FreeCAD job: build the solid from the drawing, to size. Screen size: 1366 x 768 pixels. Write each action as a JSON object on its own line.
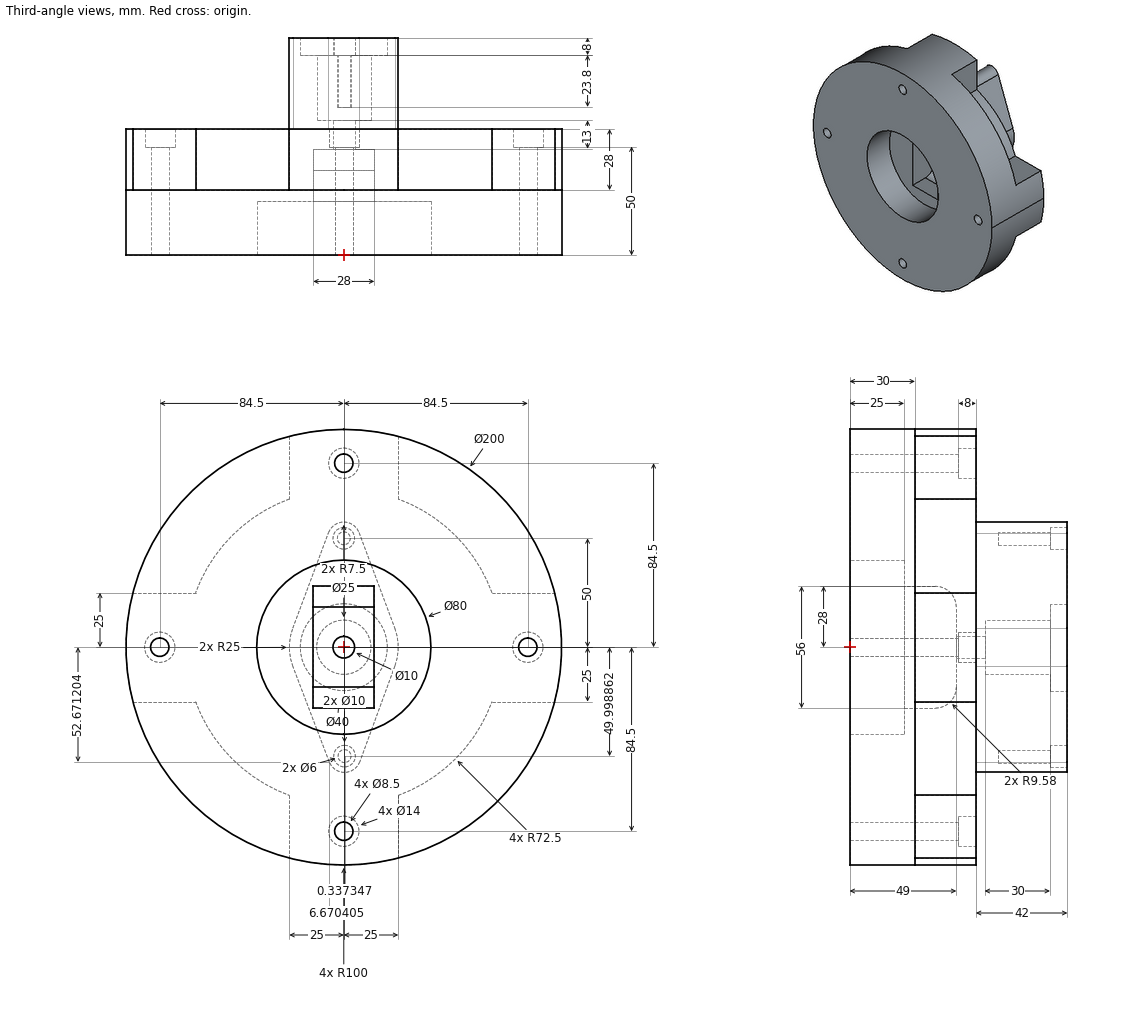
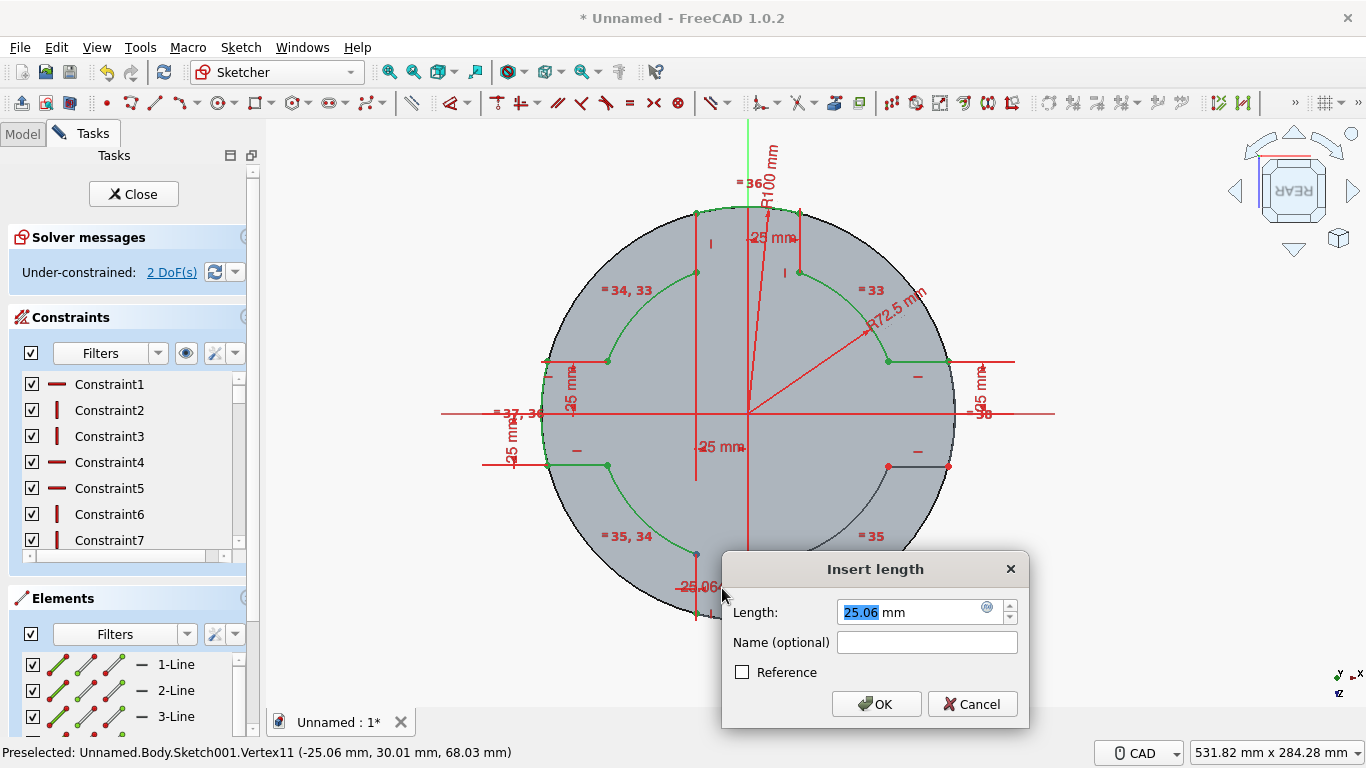
{"action": "type", "text": "25"}
{"action": "key", "text": "Return"}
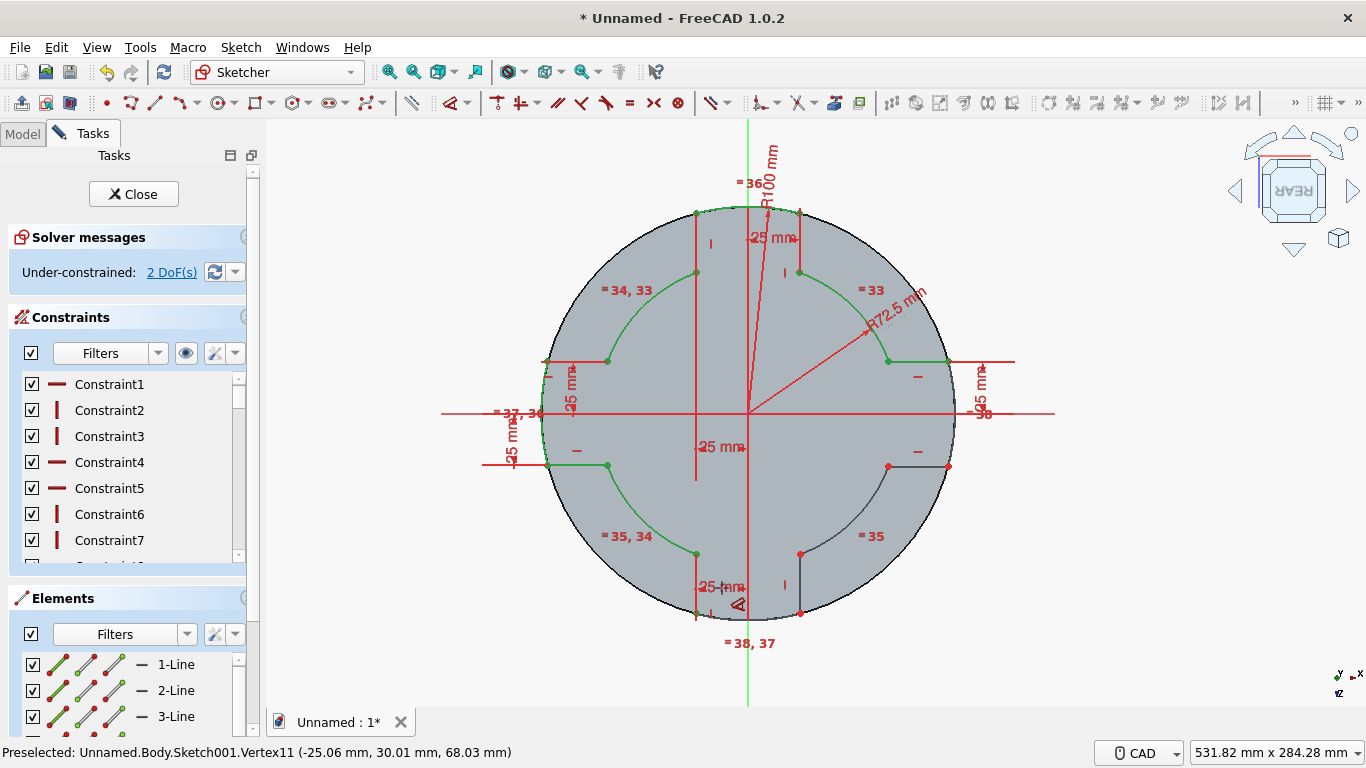
{"action": "left_click", "coordinate": [800, 614]}
{"action": "left_click", "coordinate": [774, 648]}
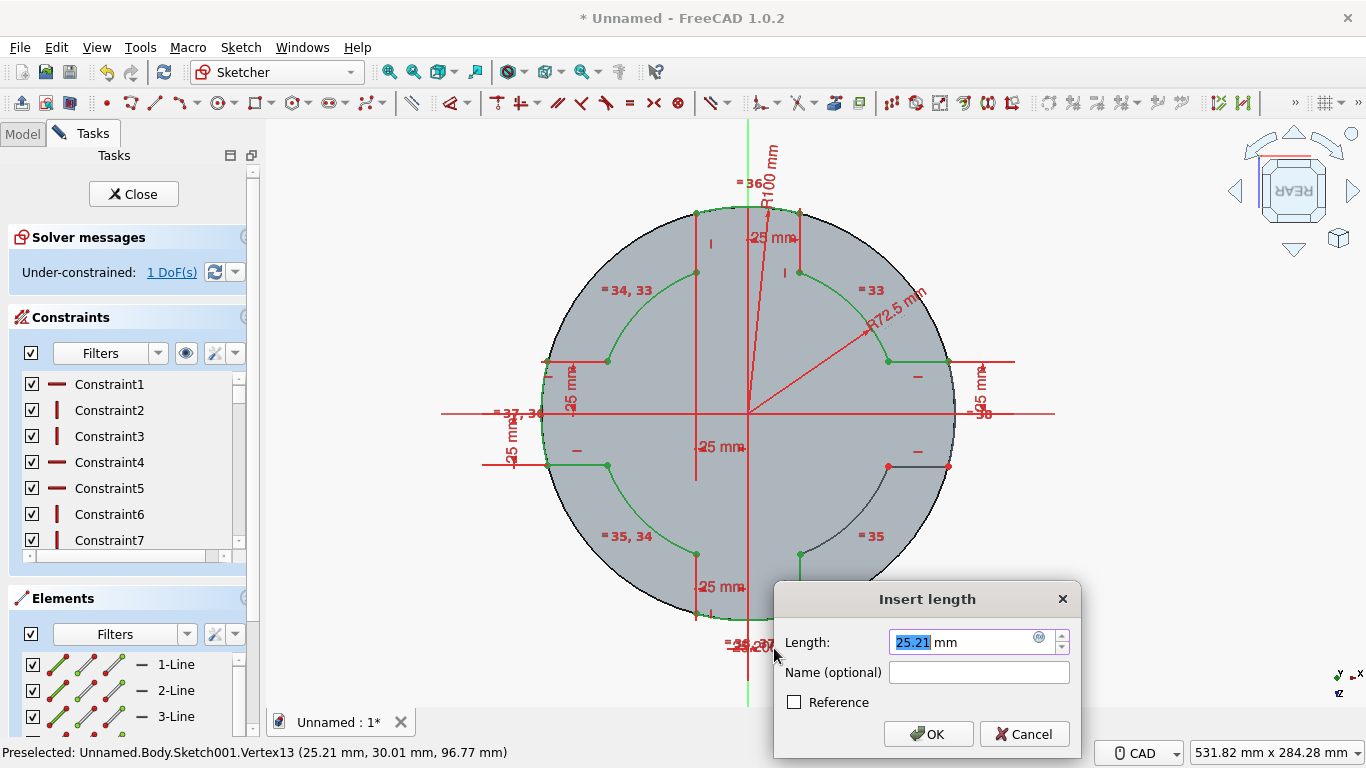
{"action": "type", "text": "25"}
{"action": "key", "text": "Return"}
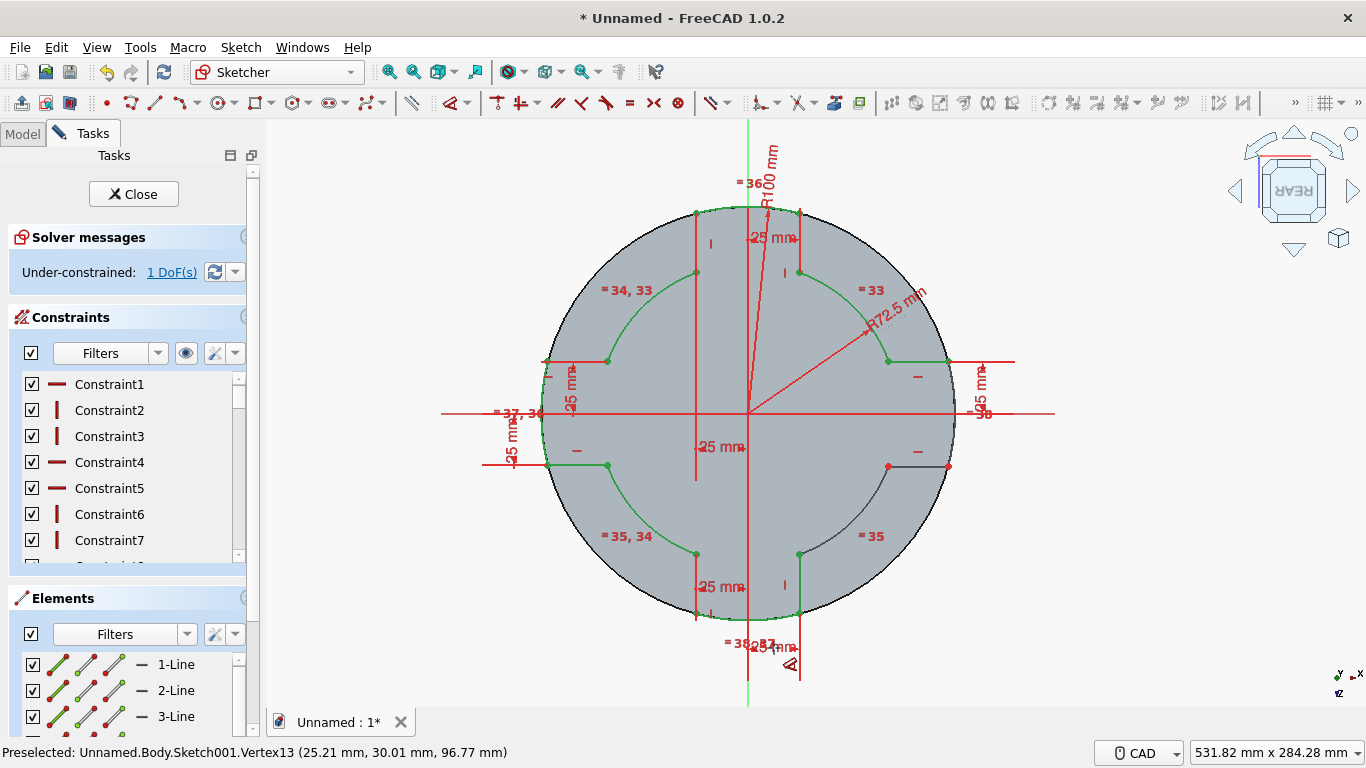
{"action": "left_click", "coordinate": [888, 467]}
{"action": "left_click", "coordinate": [922, 440]}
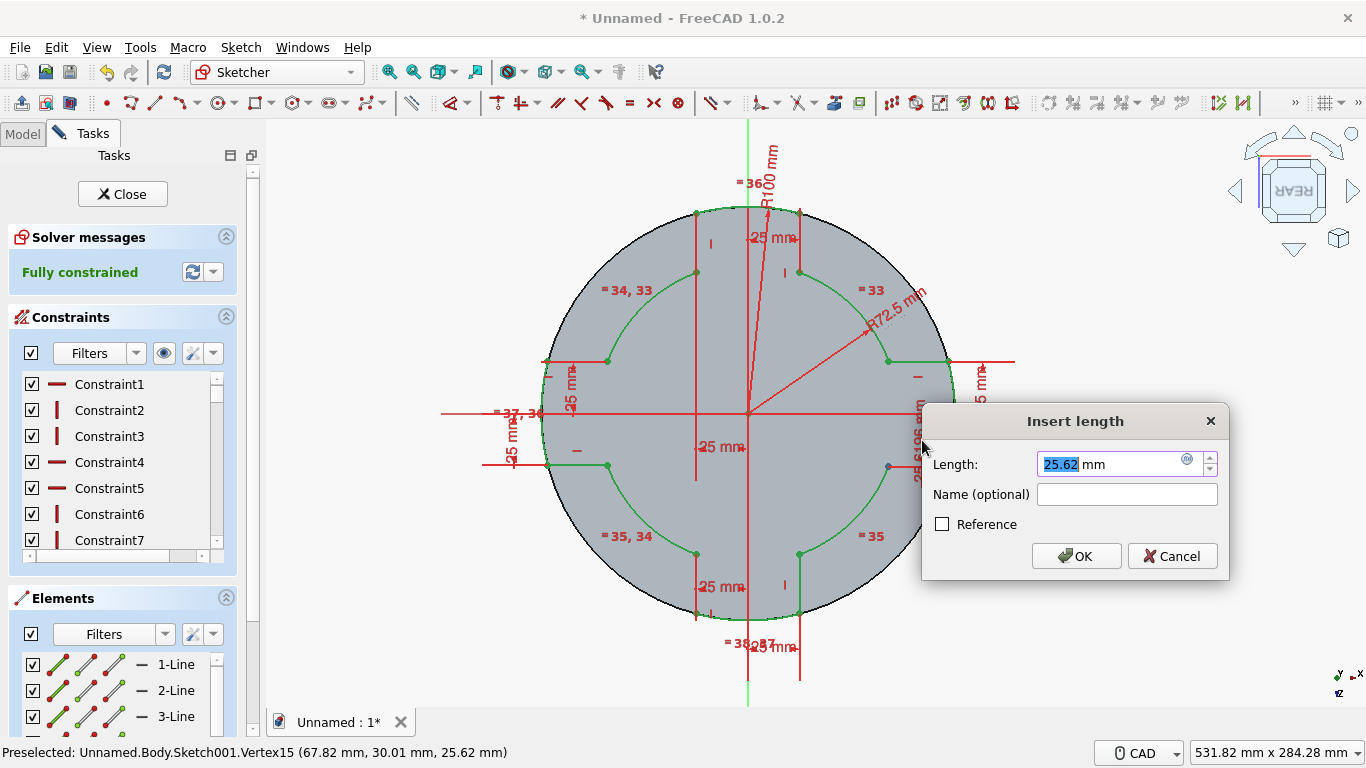
{"action": "type", "text": "25"}
{"action": "key", "text": "Return"}
{"action": "key", "text": "Escape"}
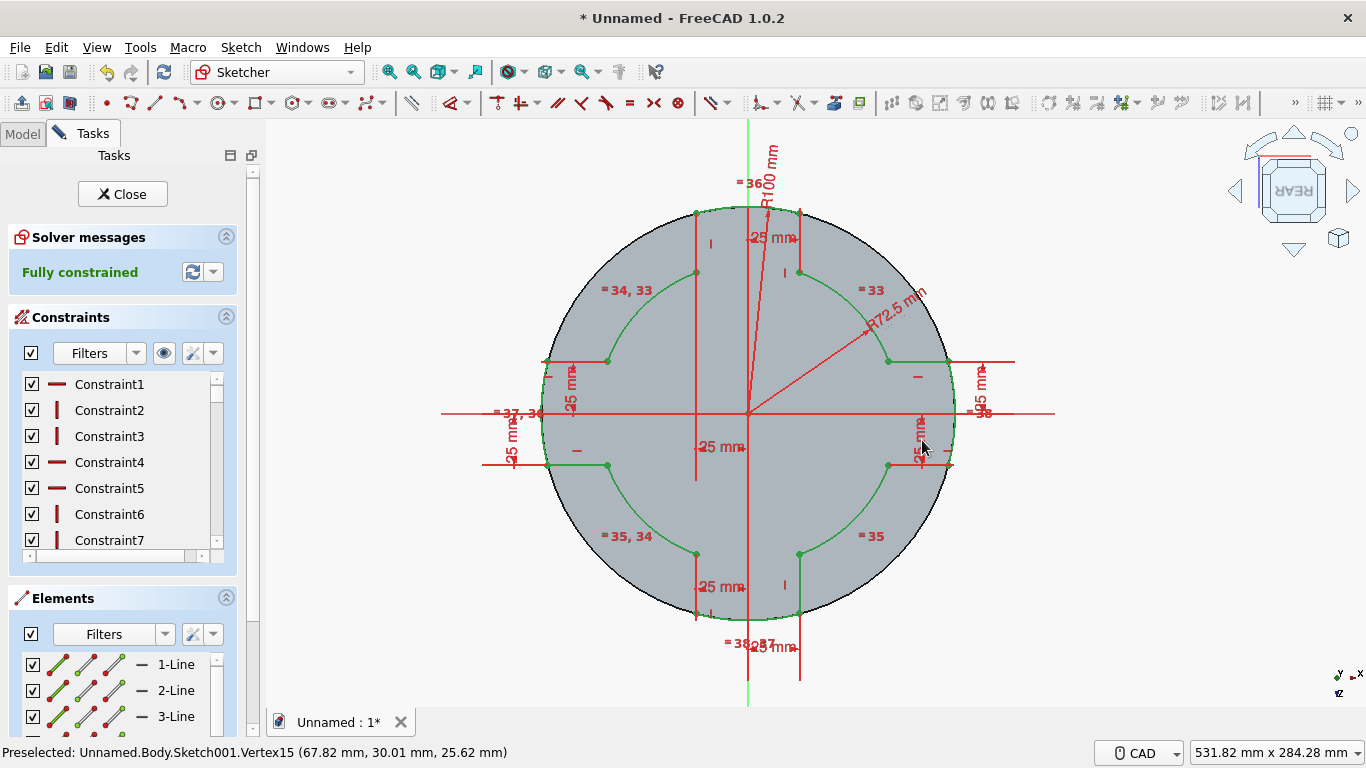
{"action": "left_click", "coordinate": [123, 194]}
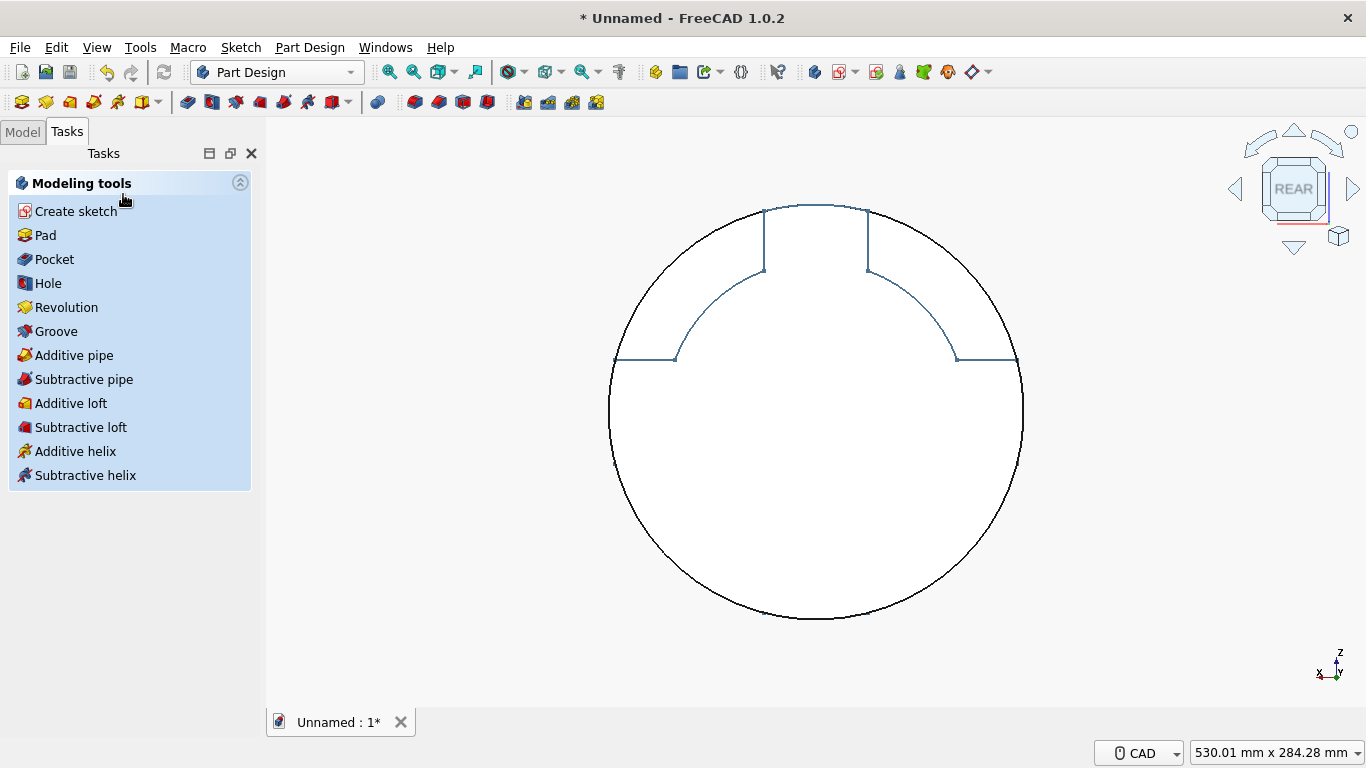
{"action": "left_click", "coordinate": [22, 102]}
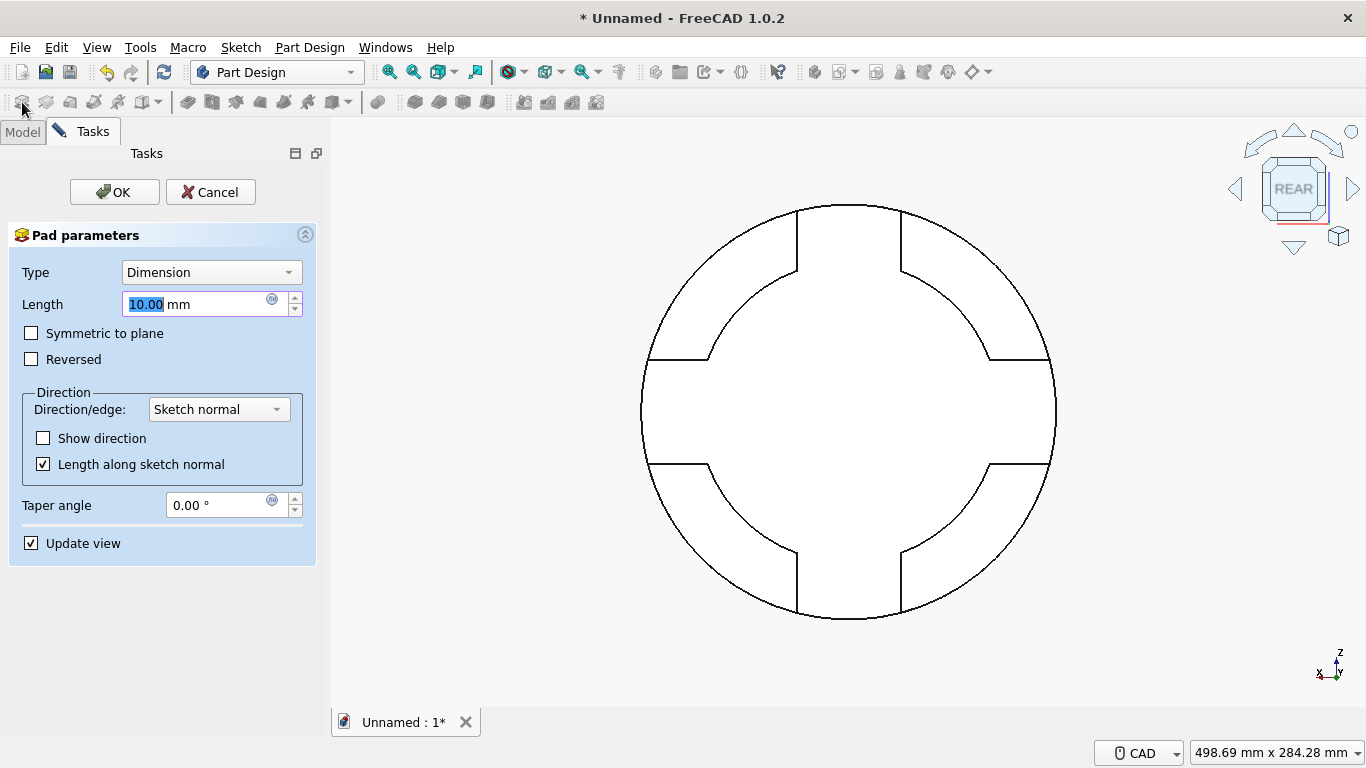
{"action": "type", "text": "28"}
{"action": "key", "text": "Tab"}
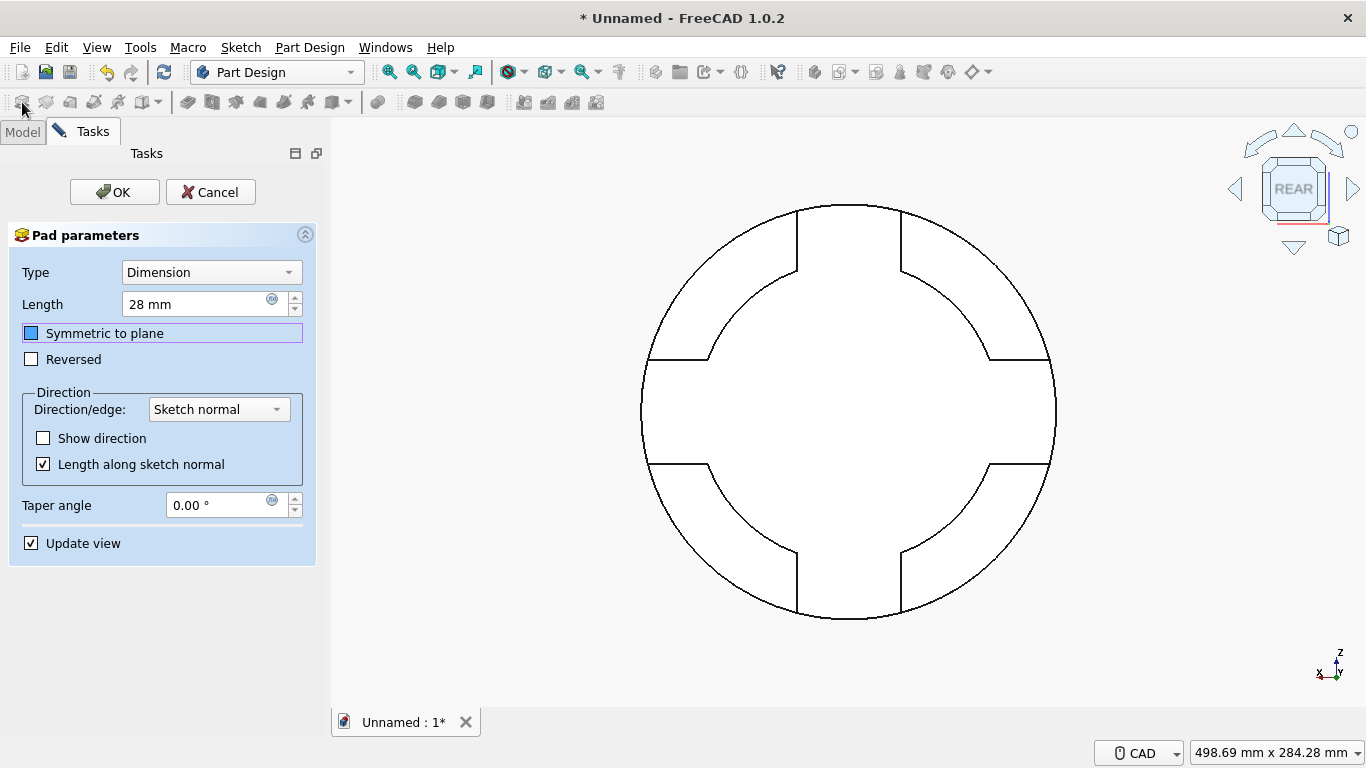
{"action": "left_click", "coordinate": [115, 192]}